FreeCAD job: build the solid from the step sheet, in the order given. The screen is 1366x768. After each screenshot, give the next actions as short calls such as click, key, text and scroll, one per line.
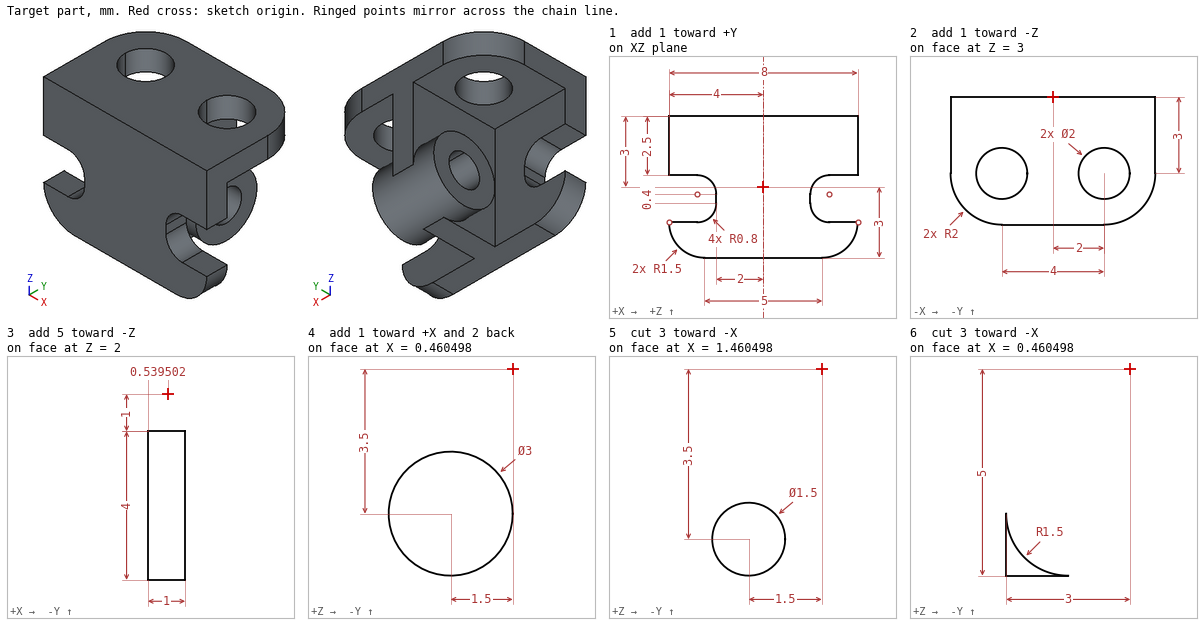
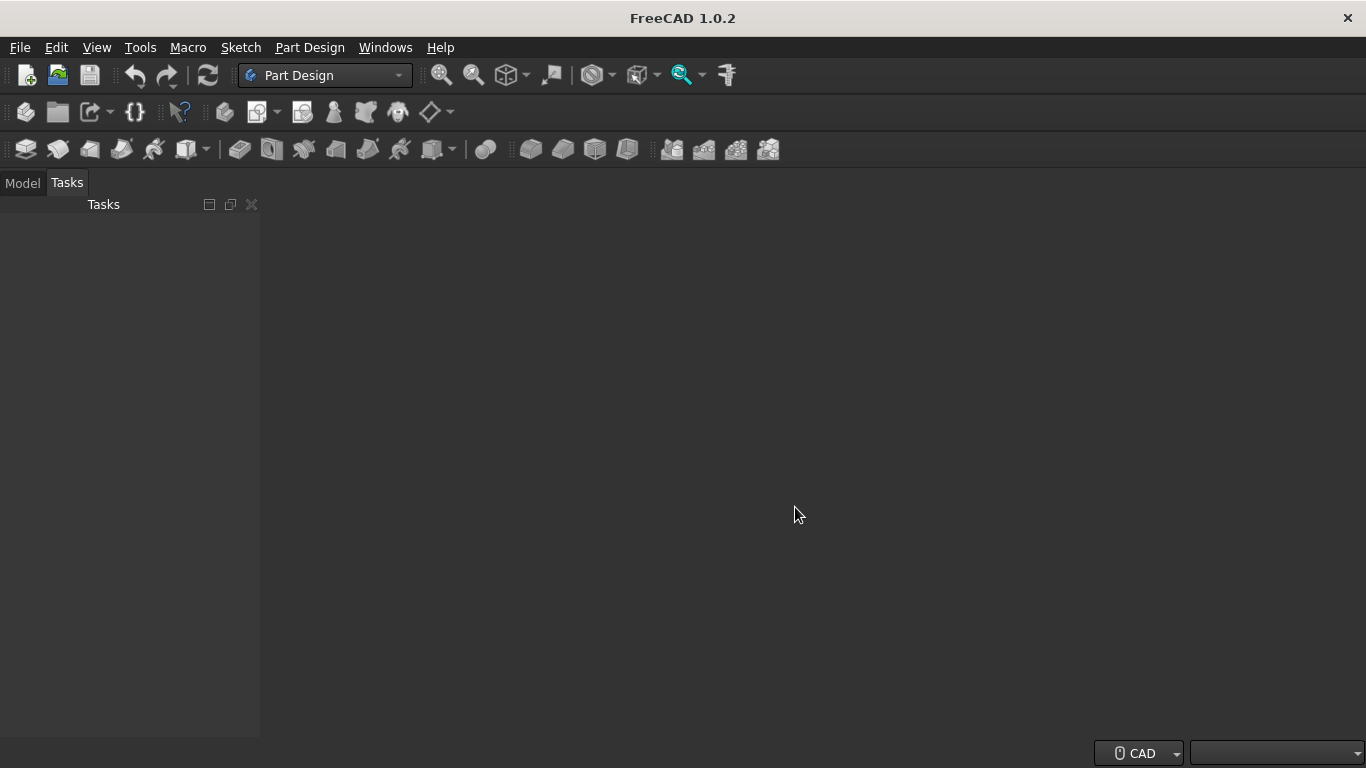
click(26, 76)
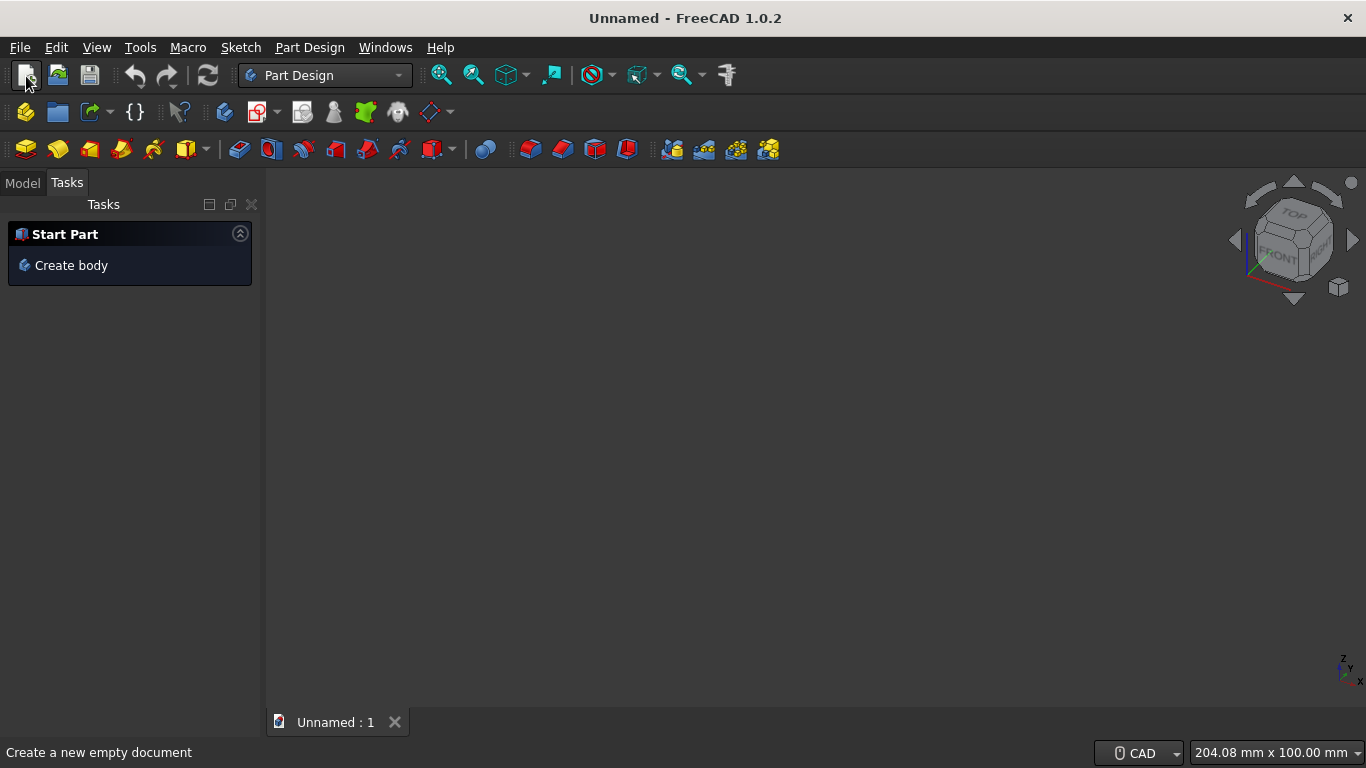
click(258, 112)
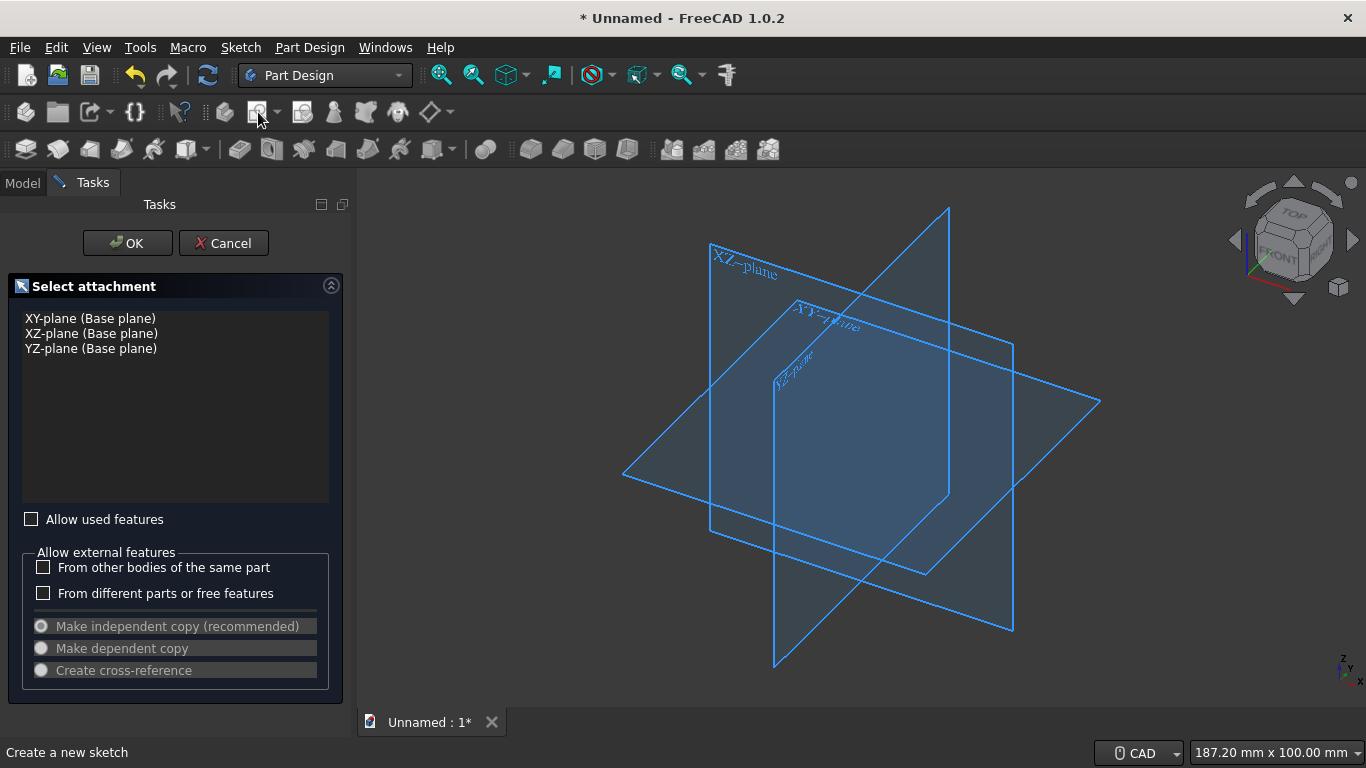
click(82, 334)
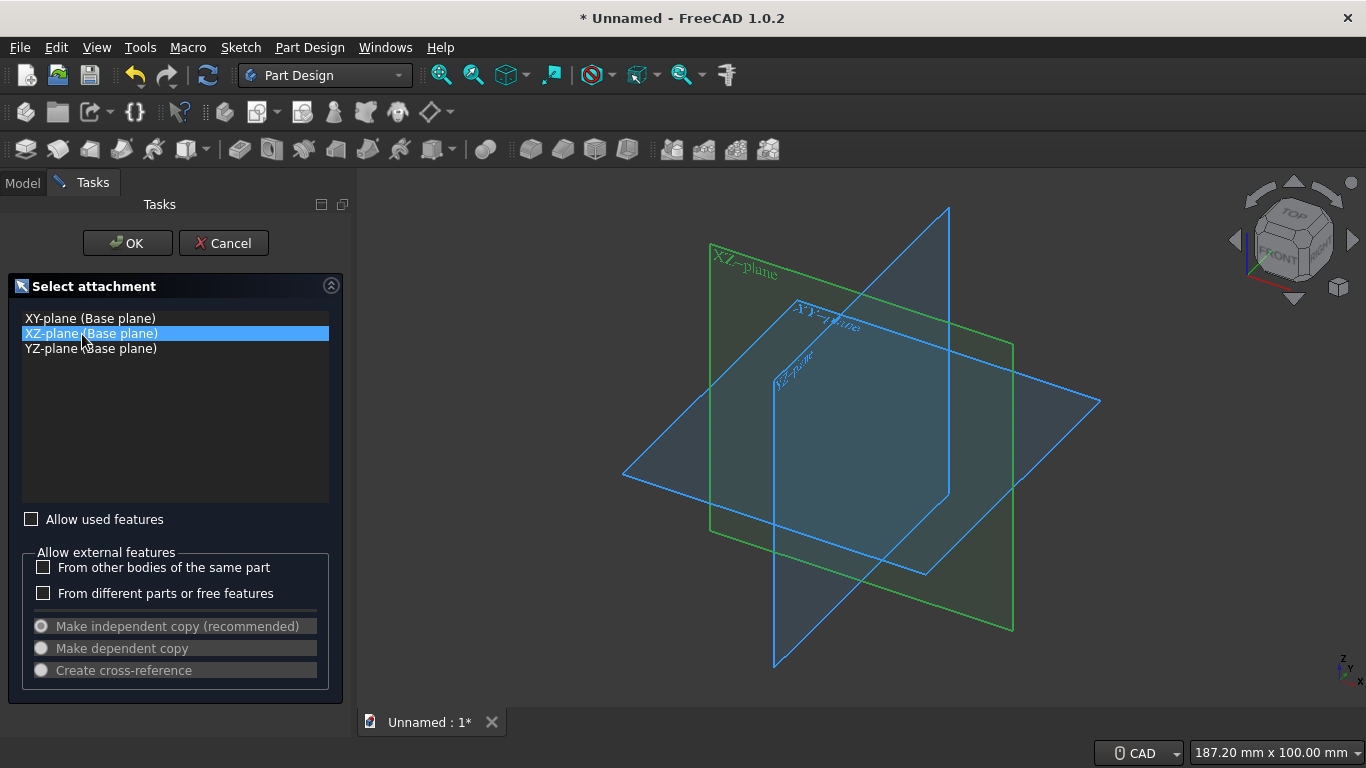
click(128, 243)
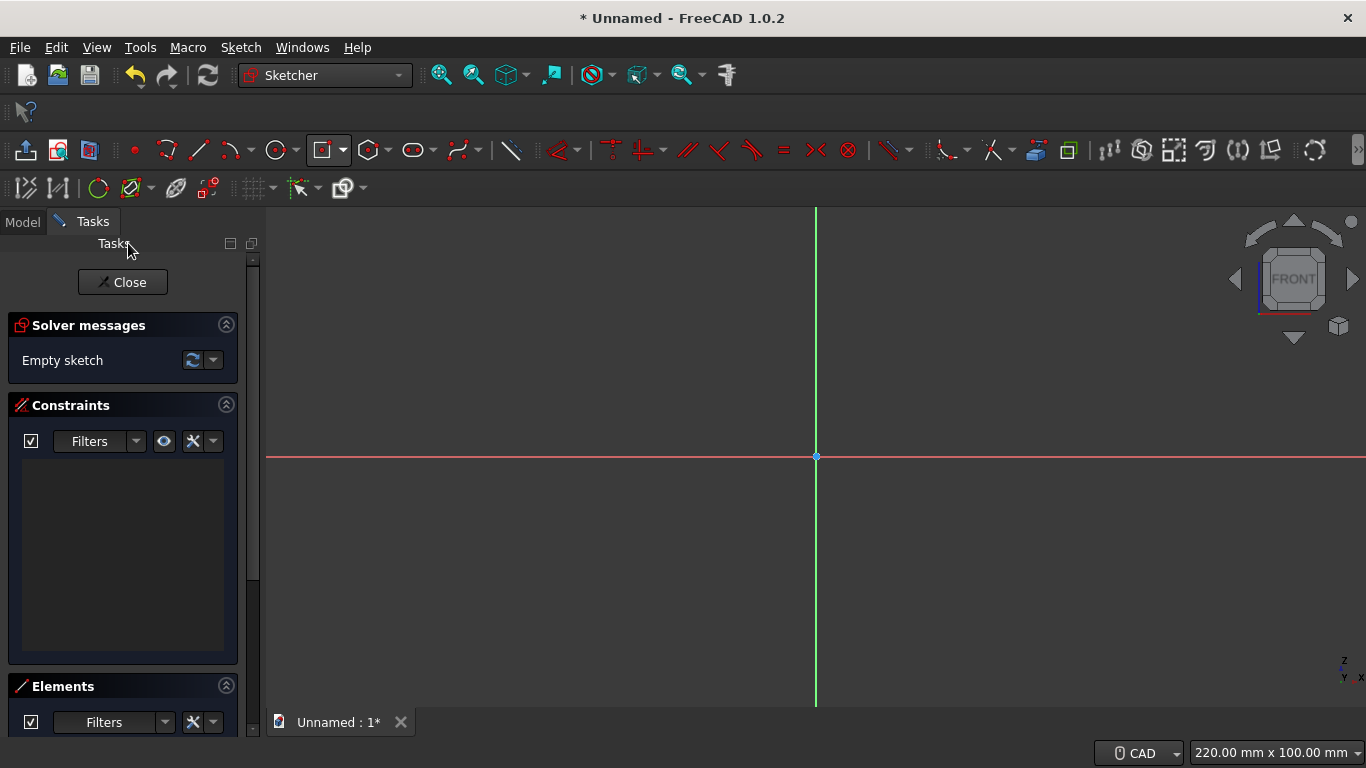
scroll(823, 457, up, 12)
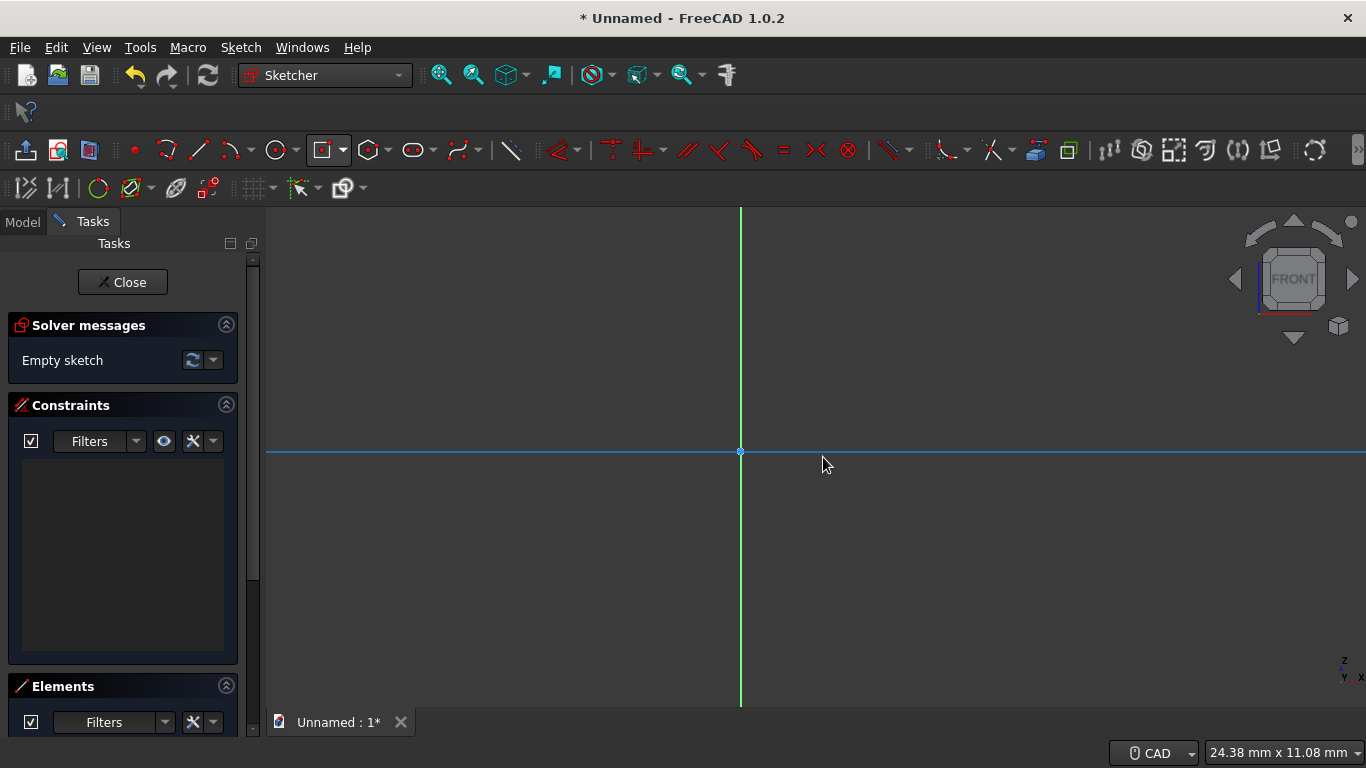
click(200, 150)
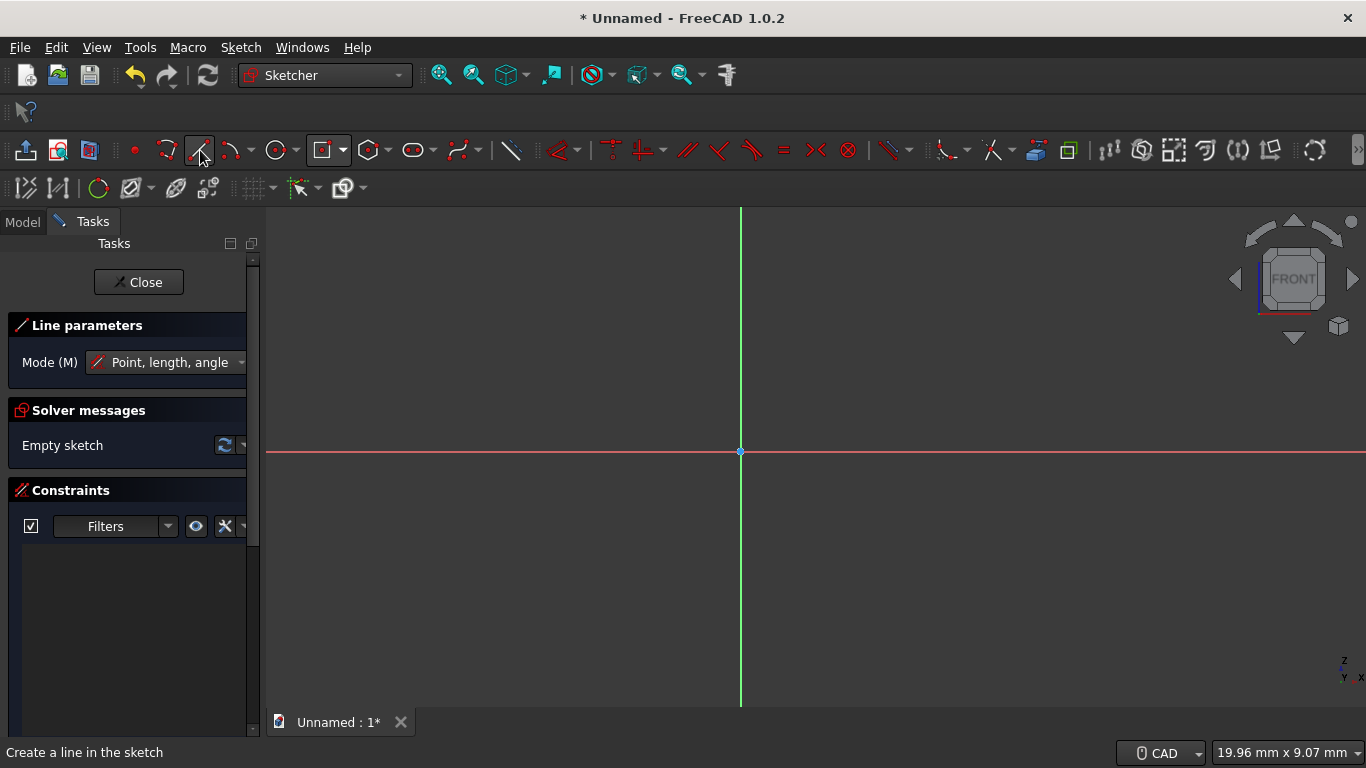
click(520, 535)
click(586, 535)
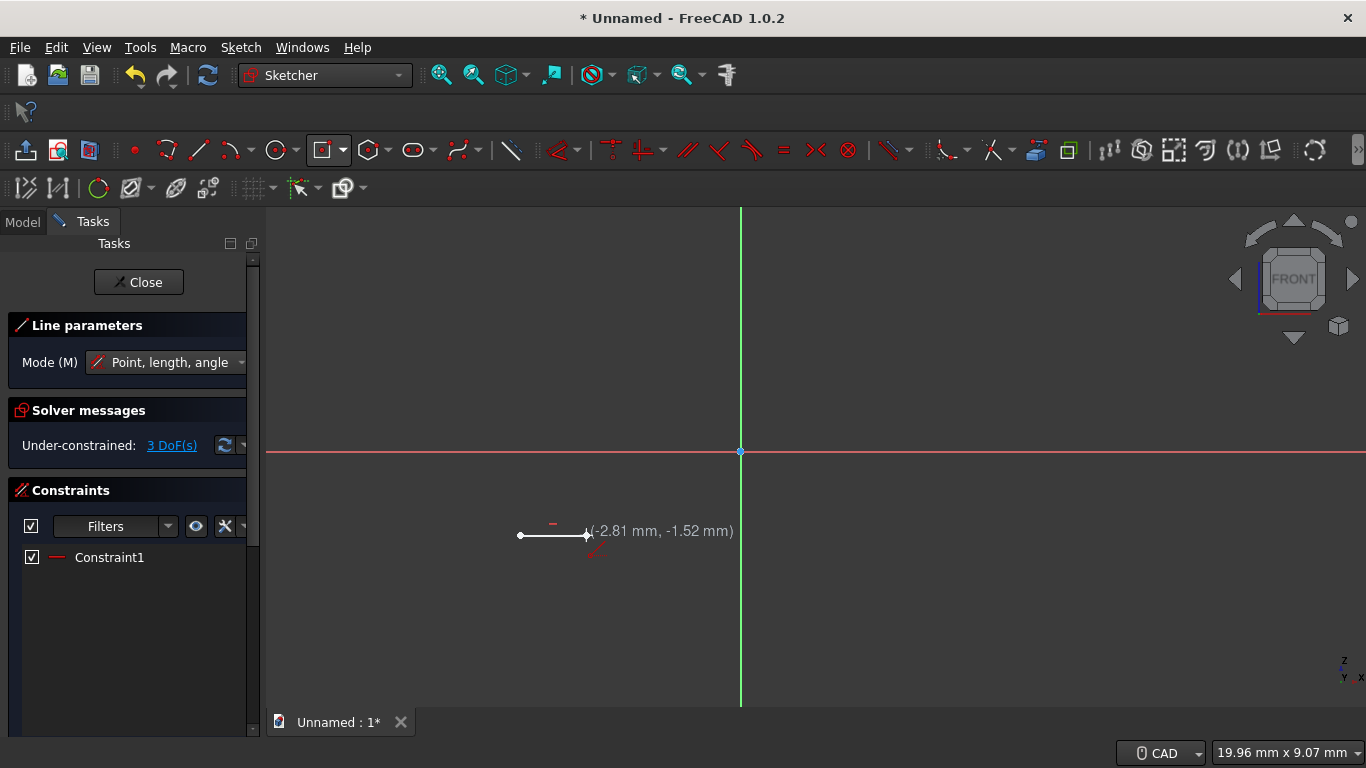
click(631, 491)
click(631, 469)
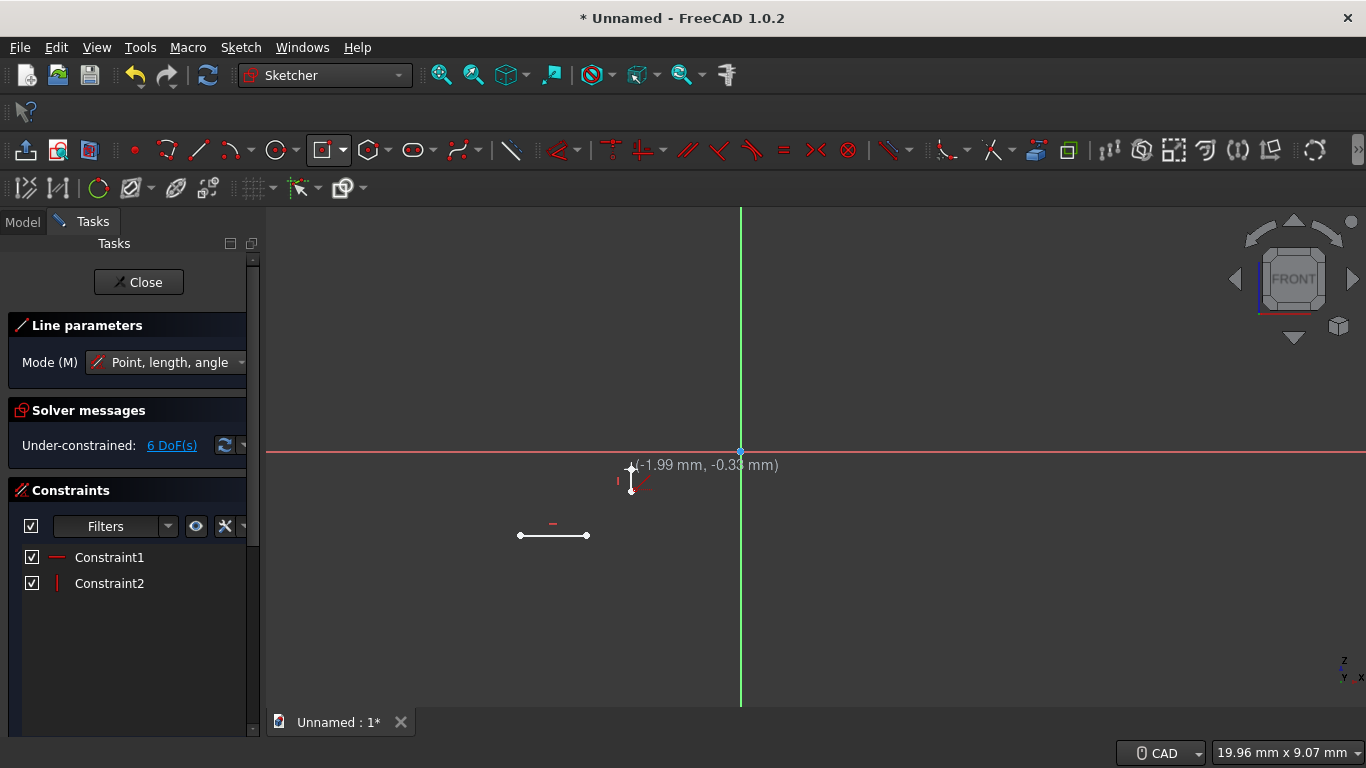
click(168, 150)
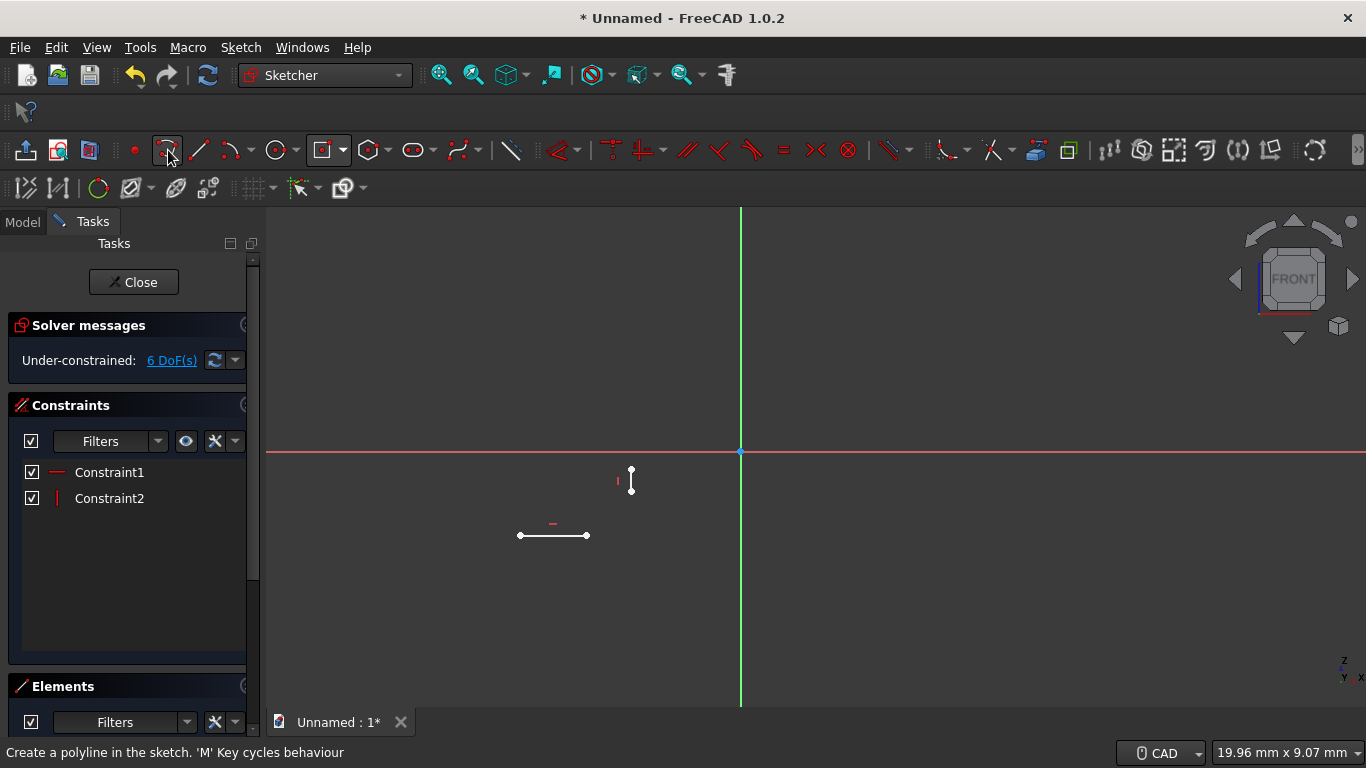
click(586, 424)
click(520, 424)
click(520, 287)
click(961, 287)
click(961, 424)
click(895, 424)
right_click(895, 424)